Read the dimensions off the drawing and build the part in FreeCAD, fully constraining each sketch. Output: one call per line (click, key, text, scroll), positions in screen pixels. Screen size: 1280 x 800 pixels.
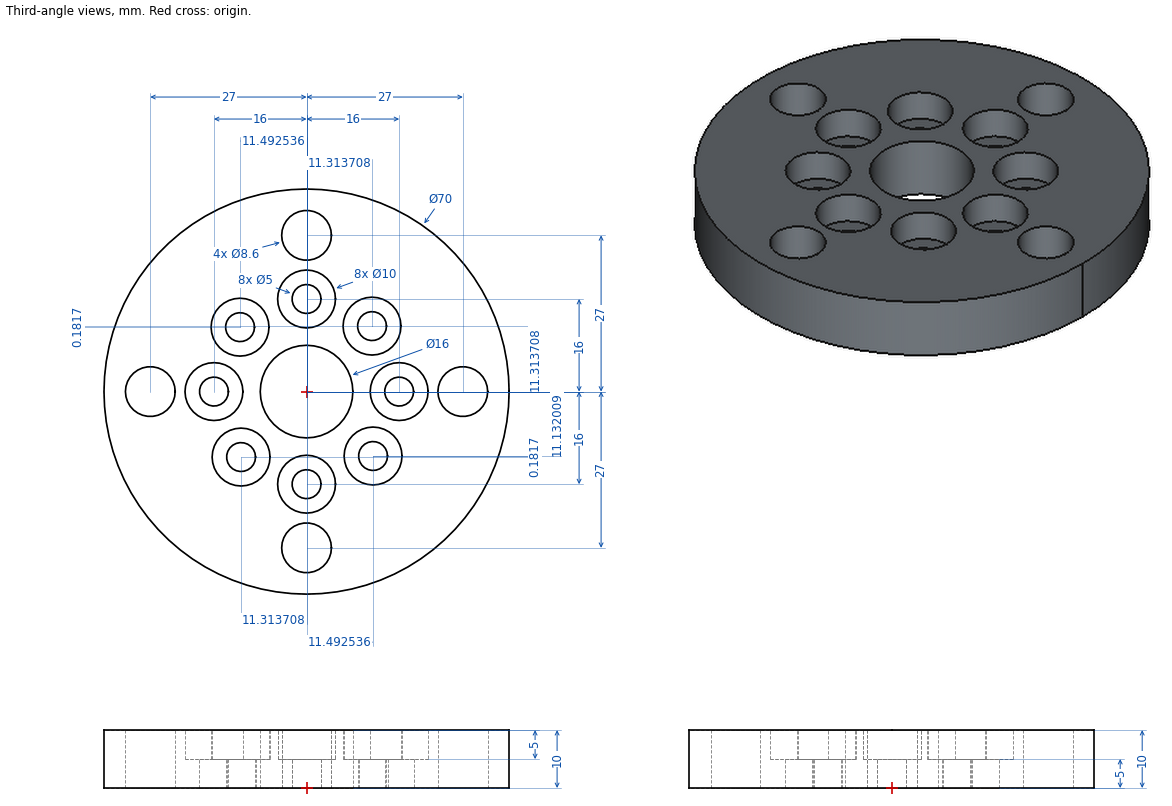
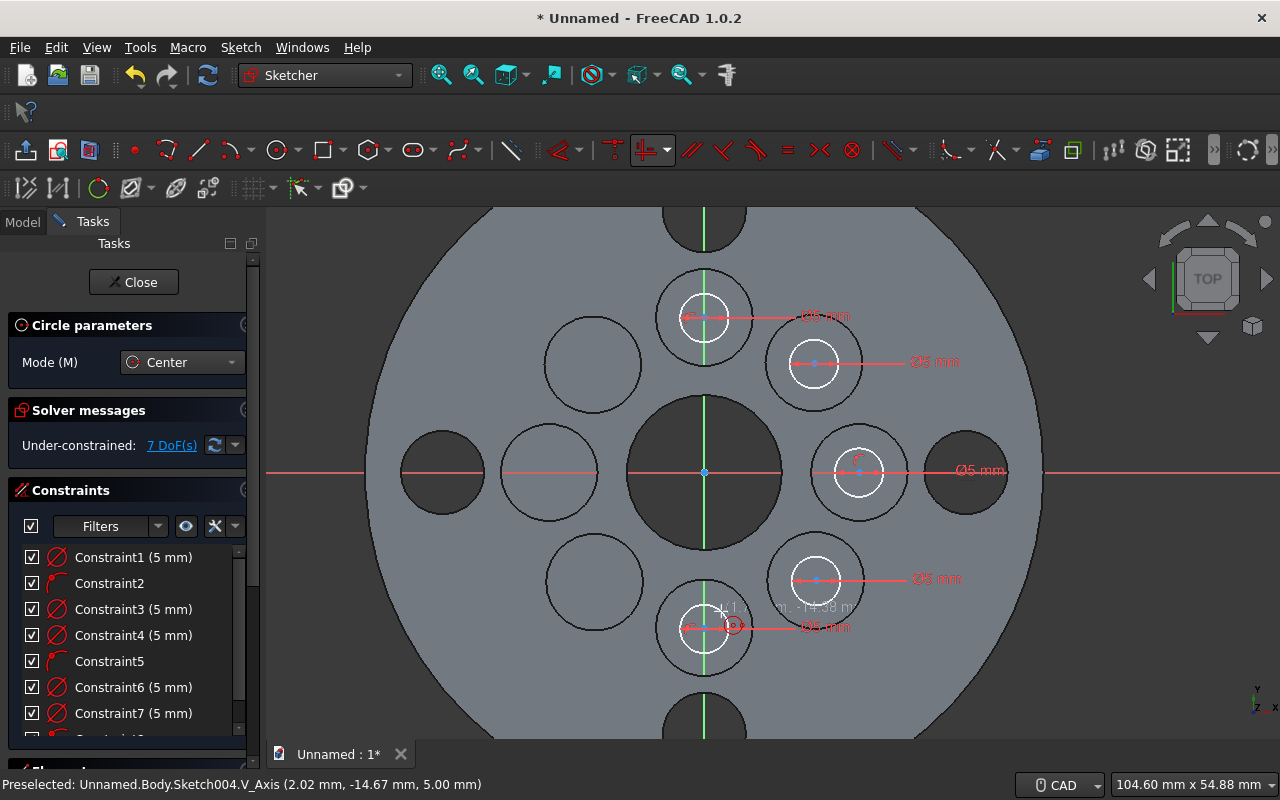
click(595, 582)
move(612, 565)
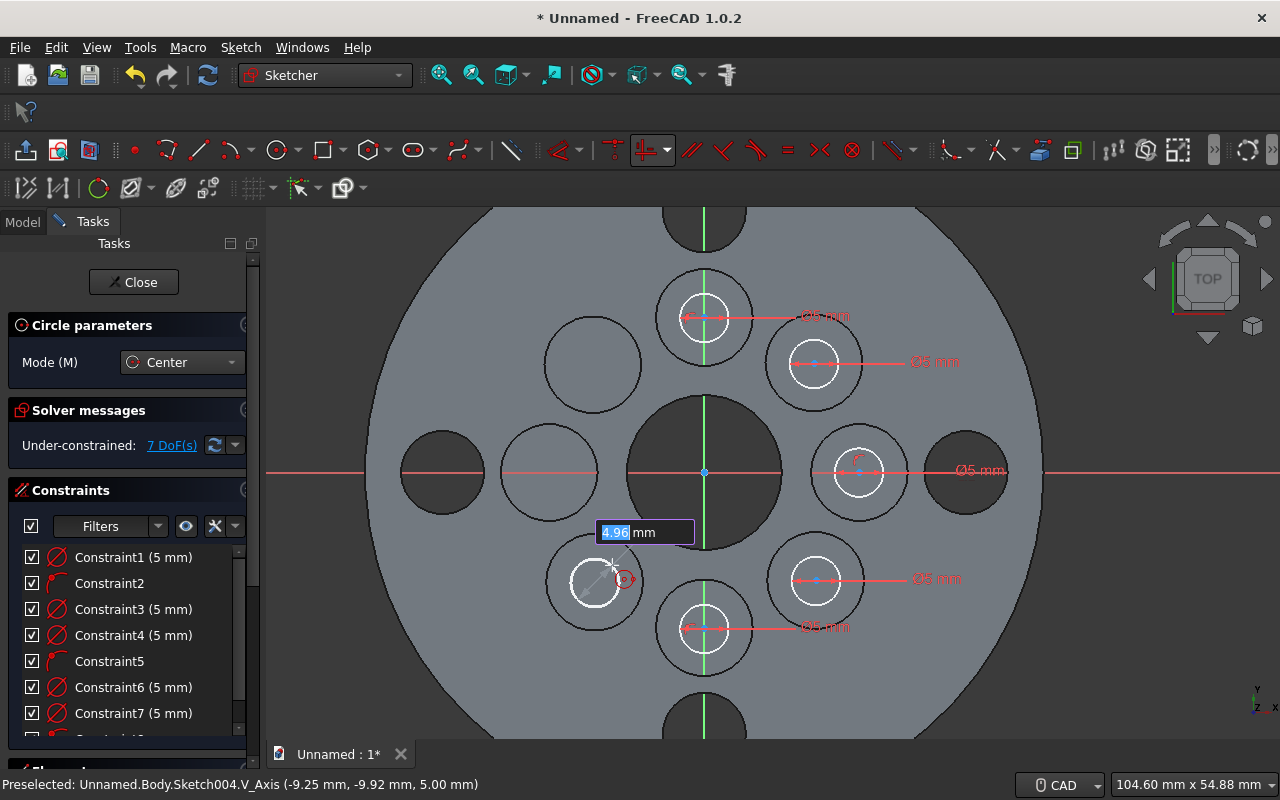
text(5)
key(Return)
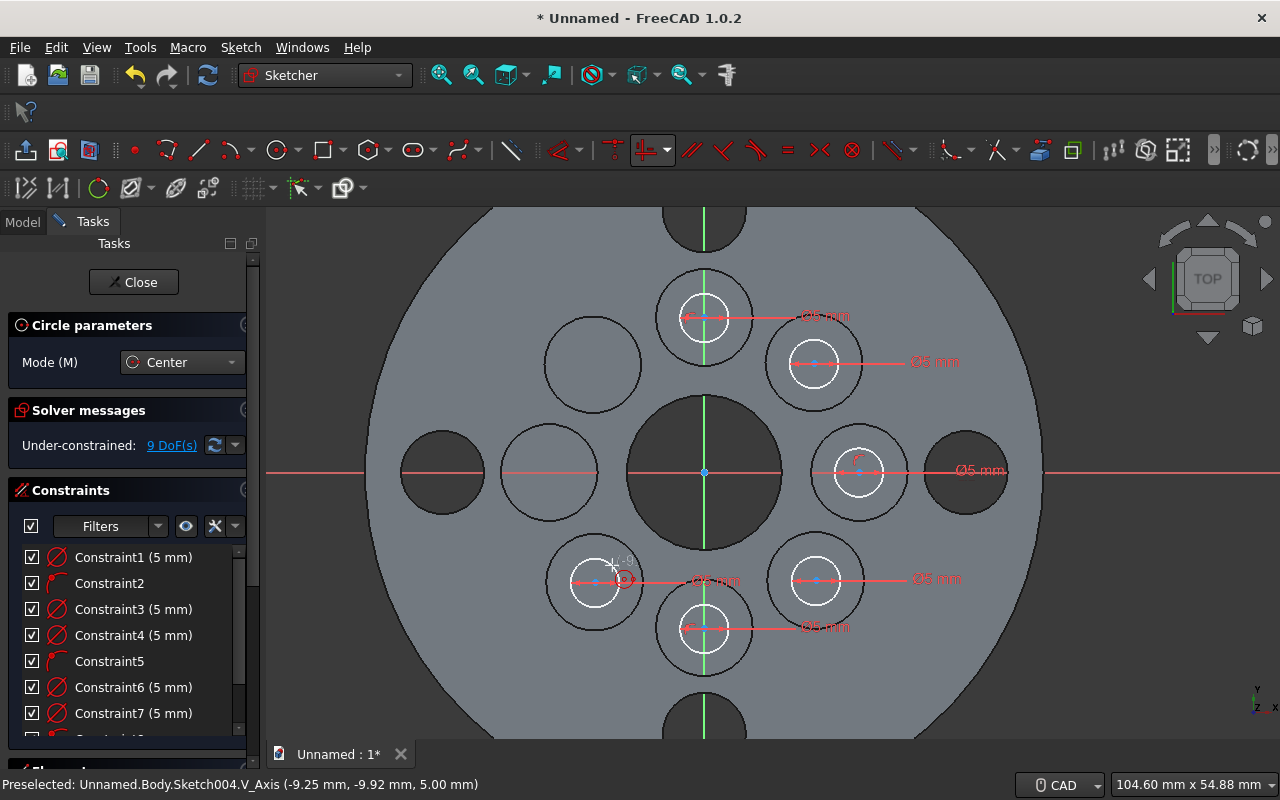
click(549, 473)
move(566, 455)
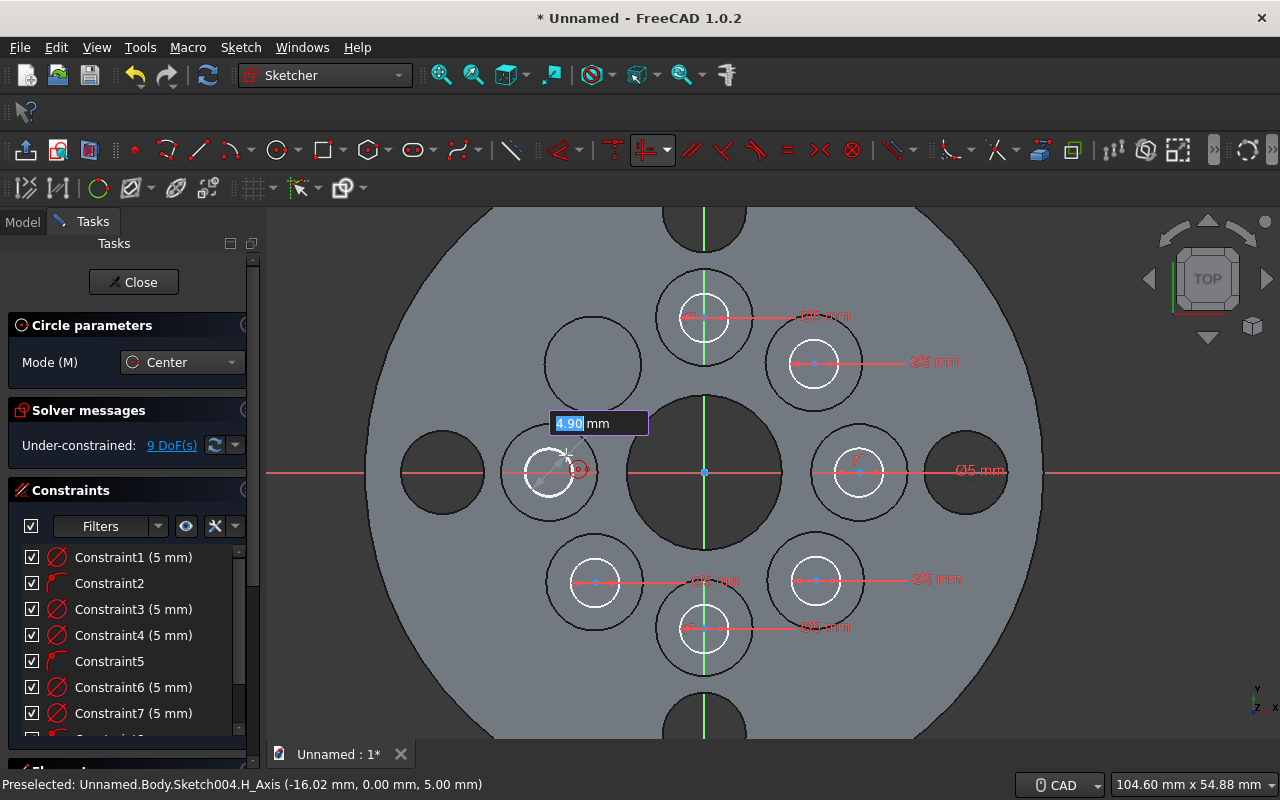
text(5)
key(Return)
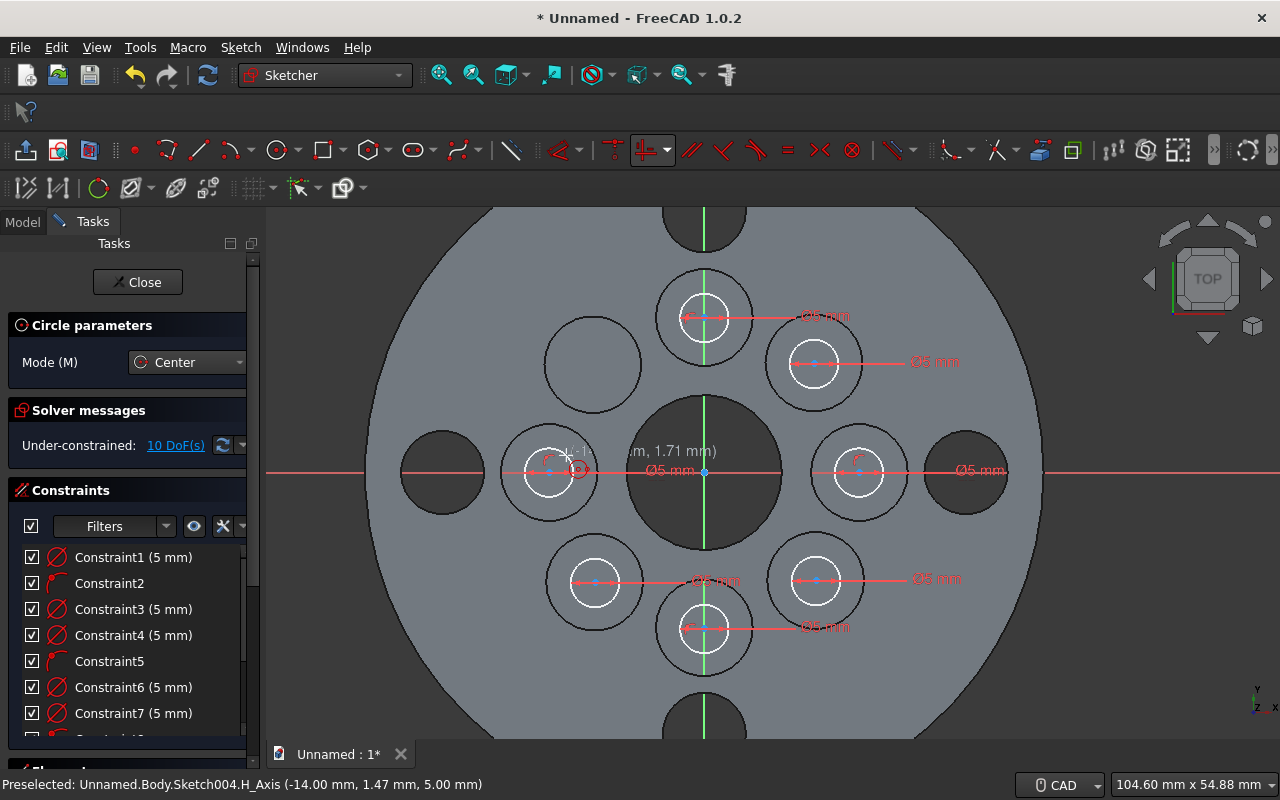
click(593, 365)
move(610, 348)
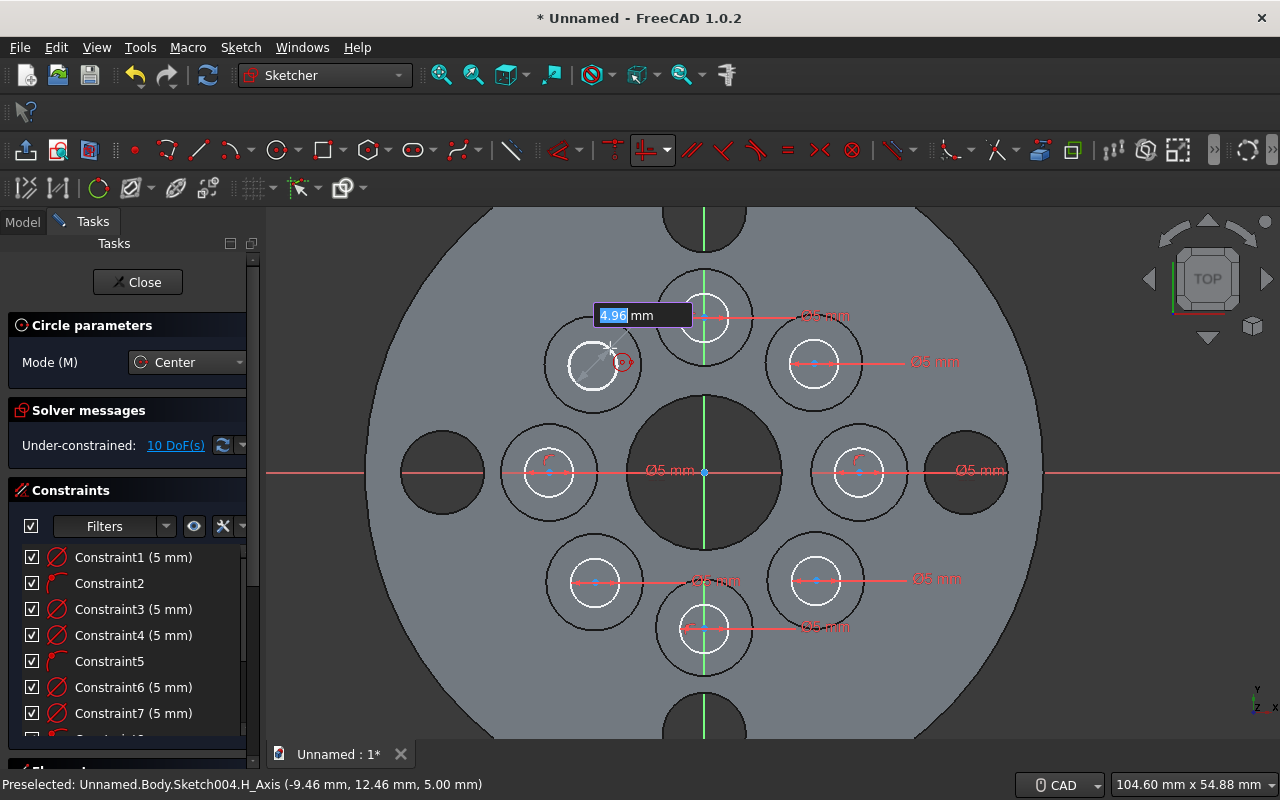
text(5)
key(Return)
key(Escape)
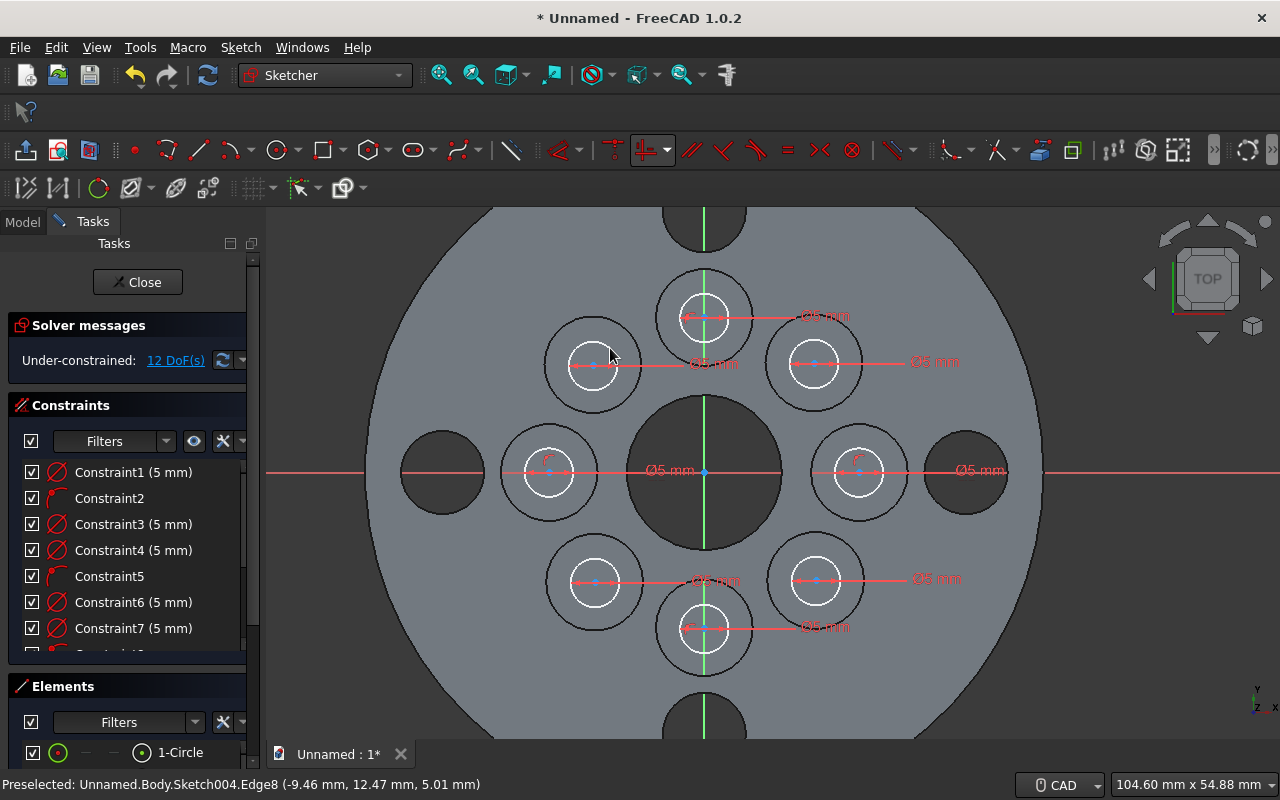
click(558, 150)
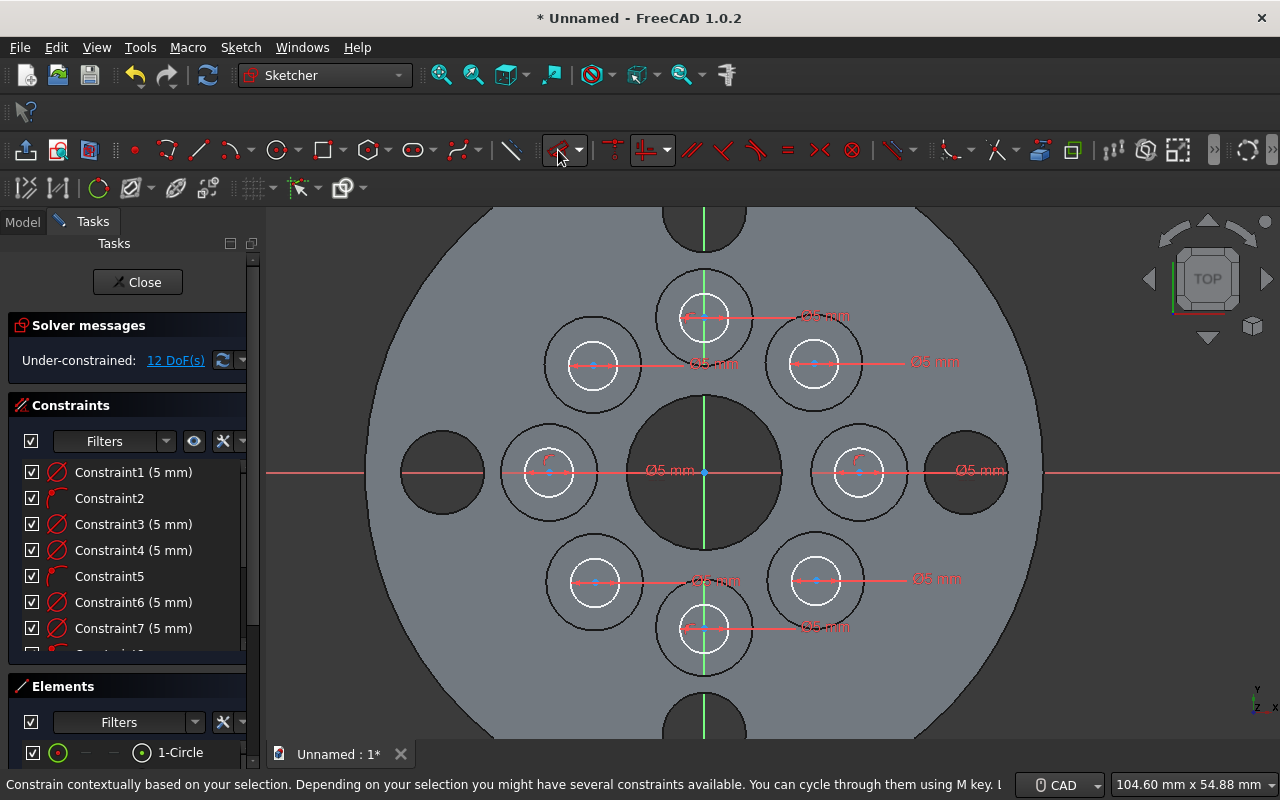
click(704, 318)
click(738, 395)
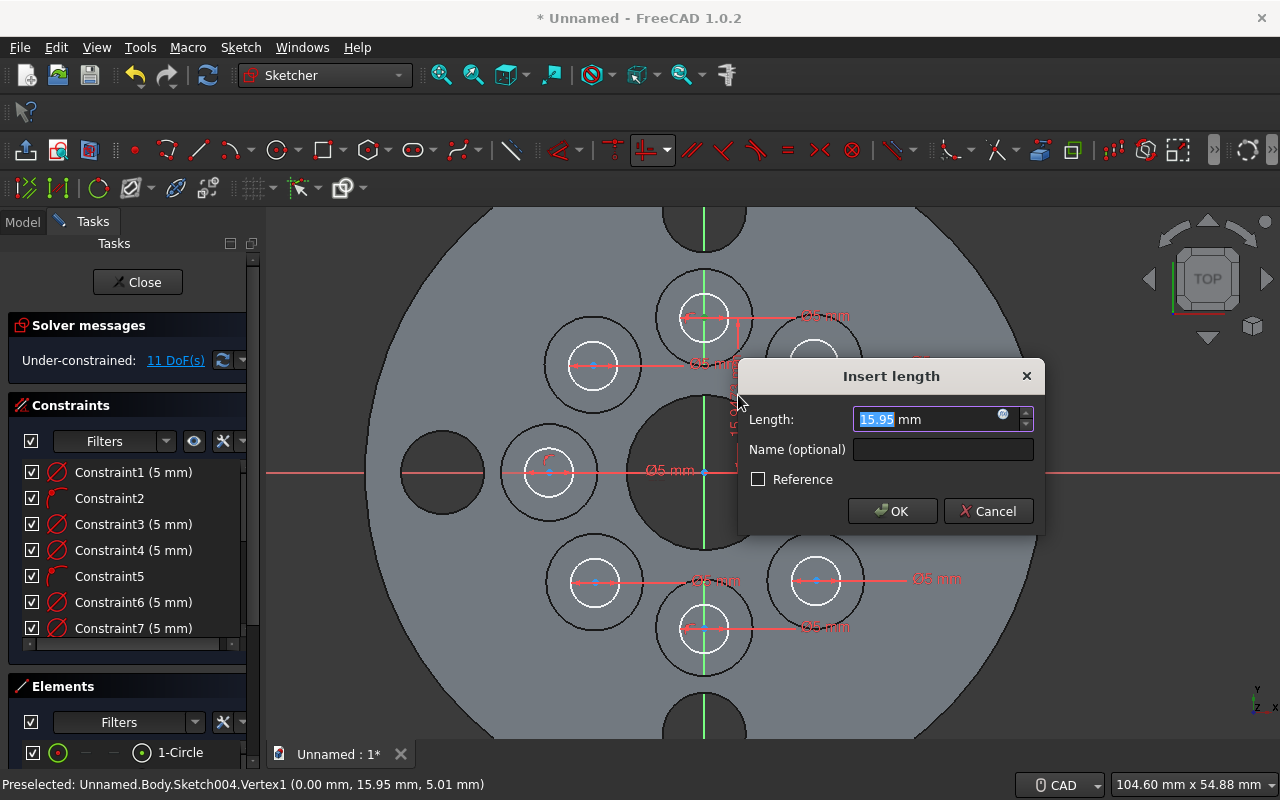
text(16)
key(Return)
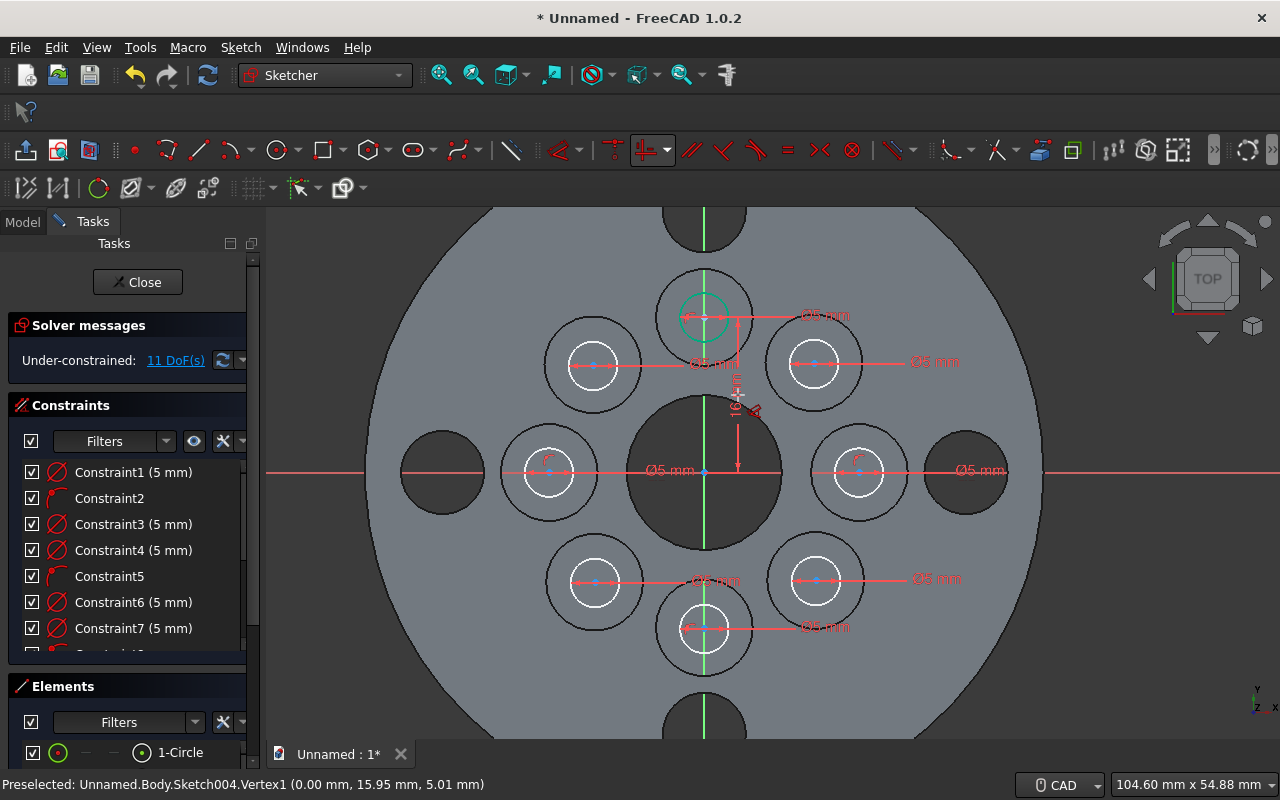
click(859, 473)
click(782, 507)